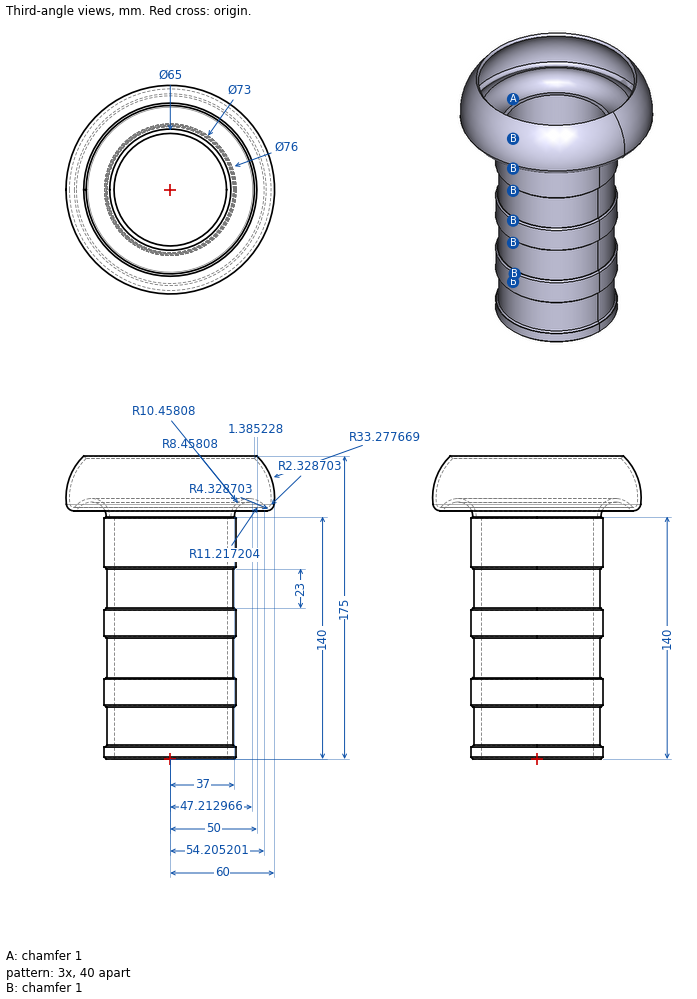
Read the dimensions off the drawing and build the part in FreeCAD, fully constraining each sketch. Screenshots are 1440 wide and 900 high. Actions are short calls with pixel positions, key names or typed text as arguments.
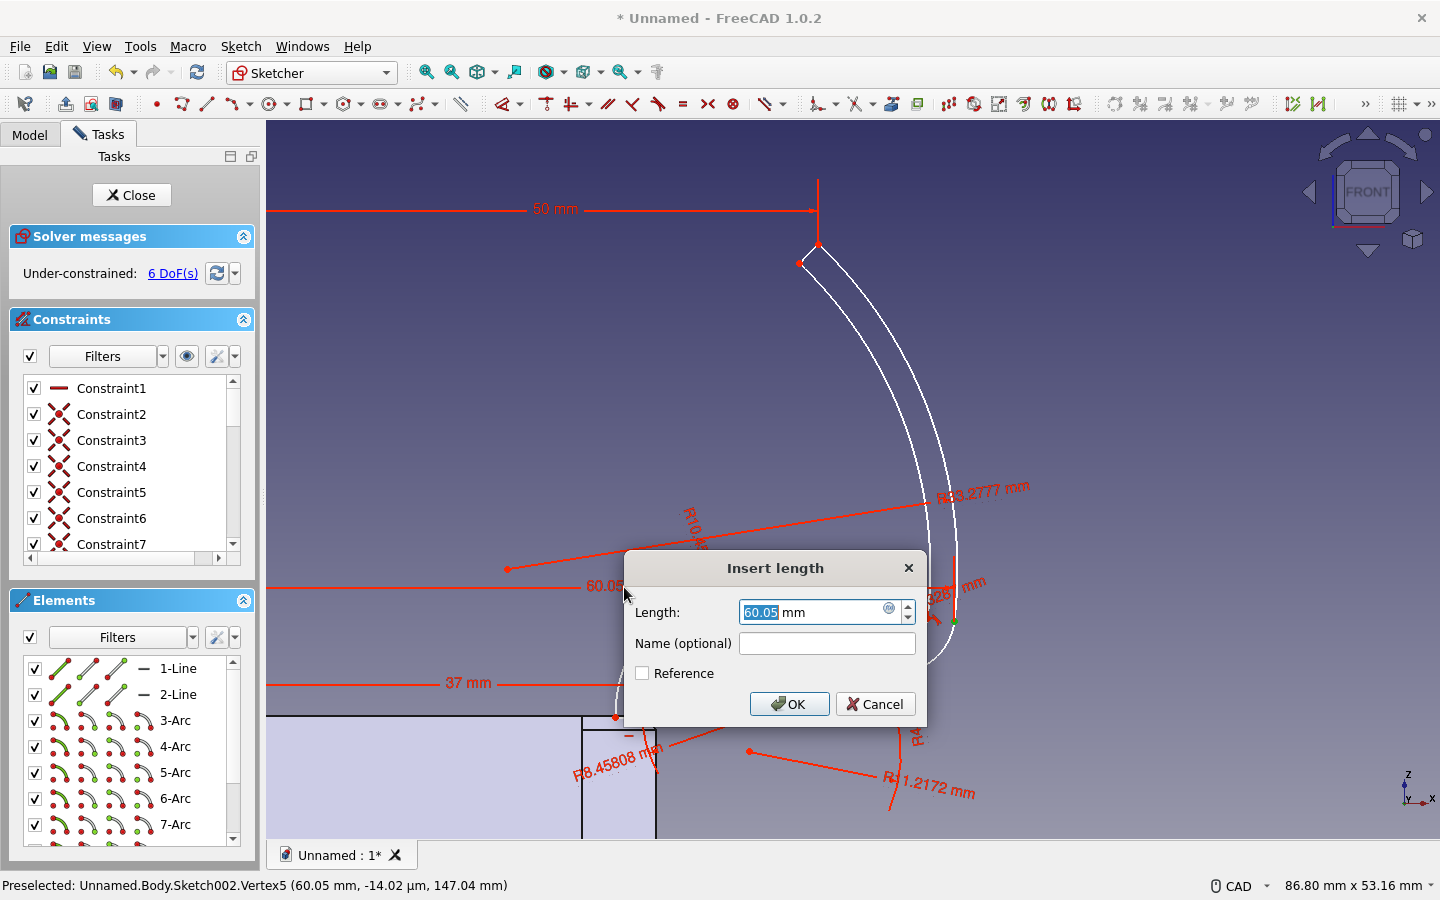
text(60)
key(Return)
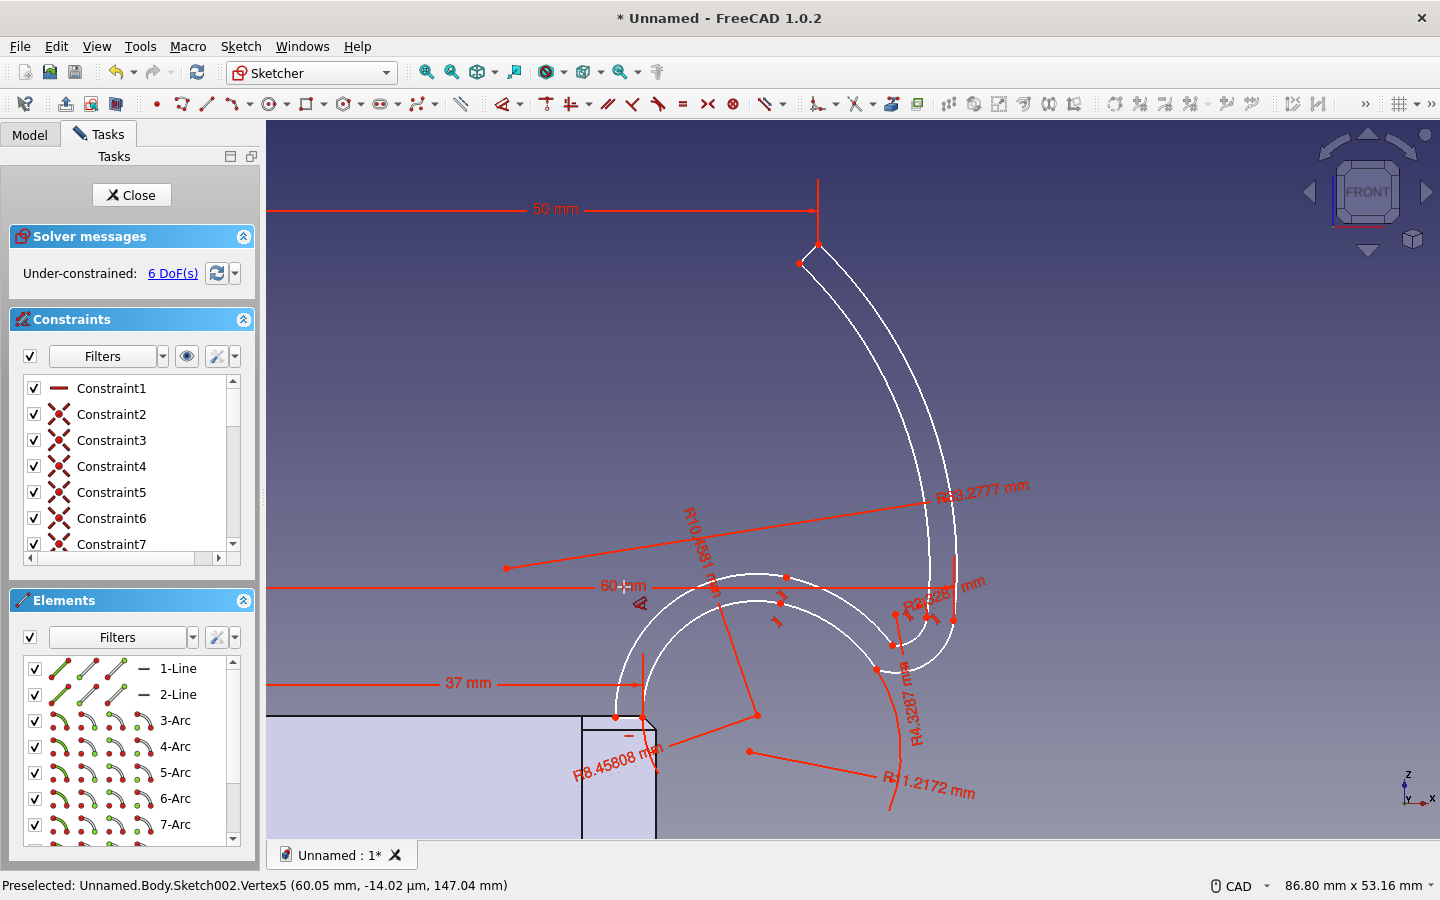
click(818, 244)
click(852, 528)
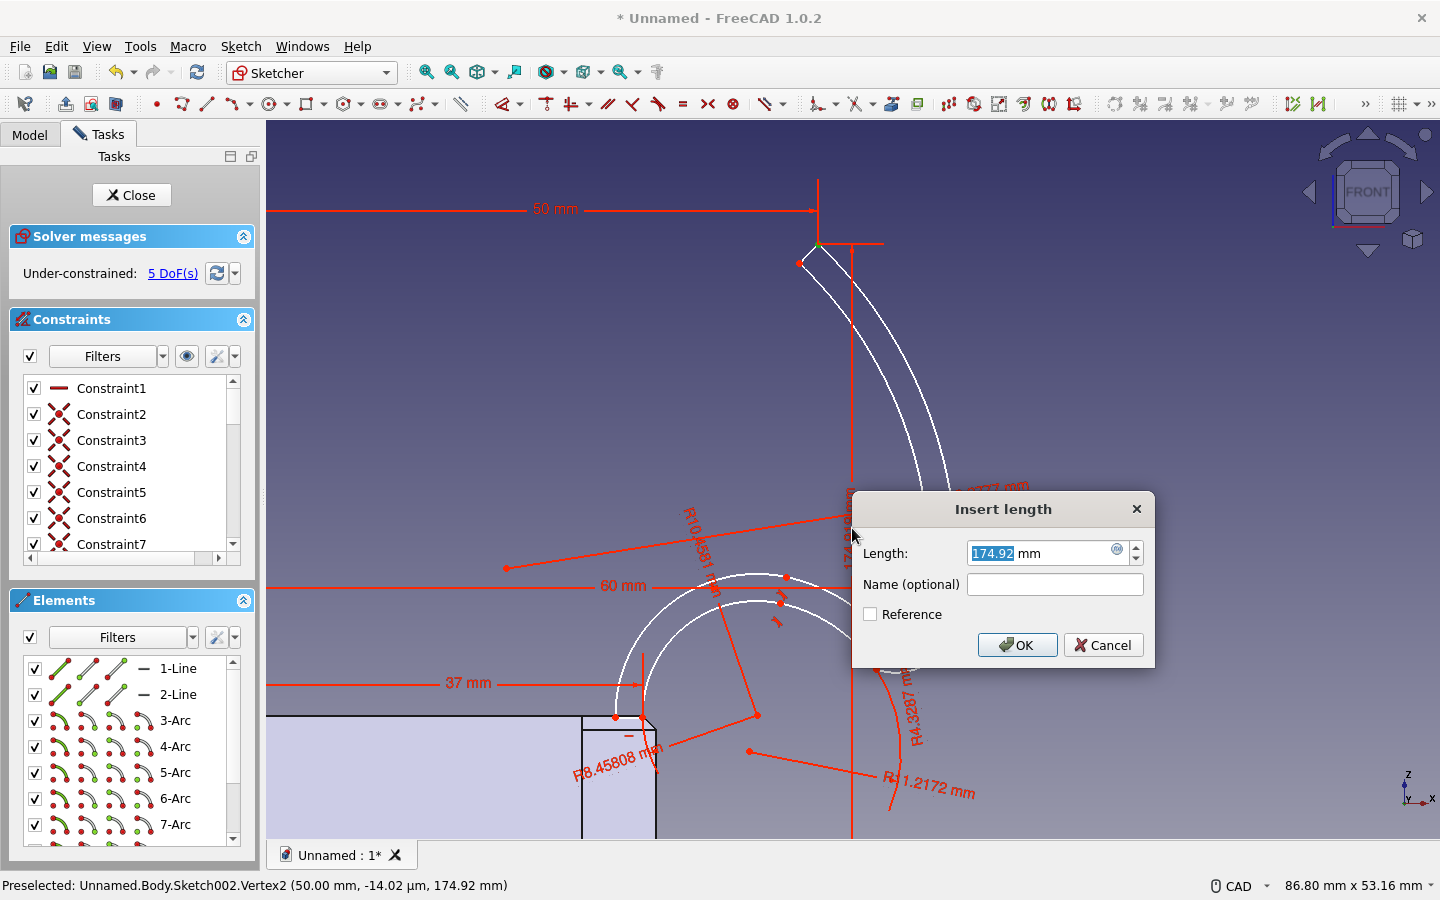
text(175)
key(Return)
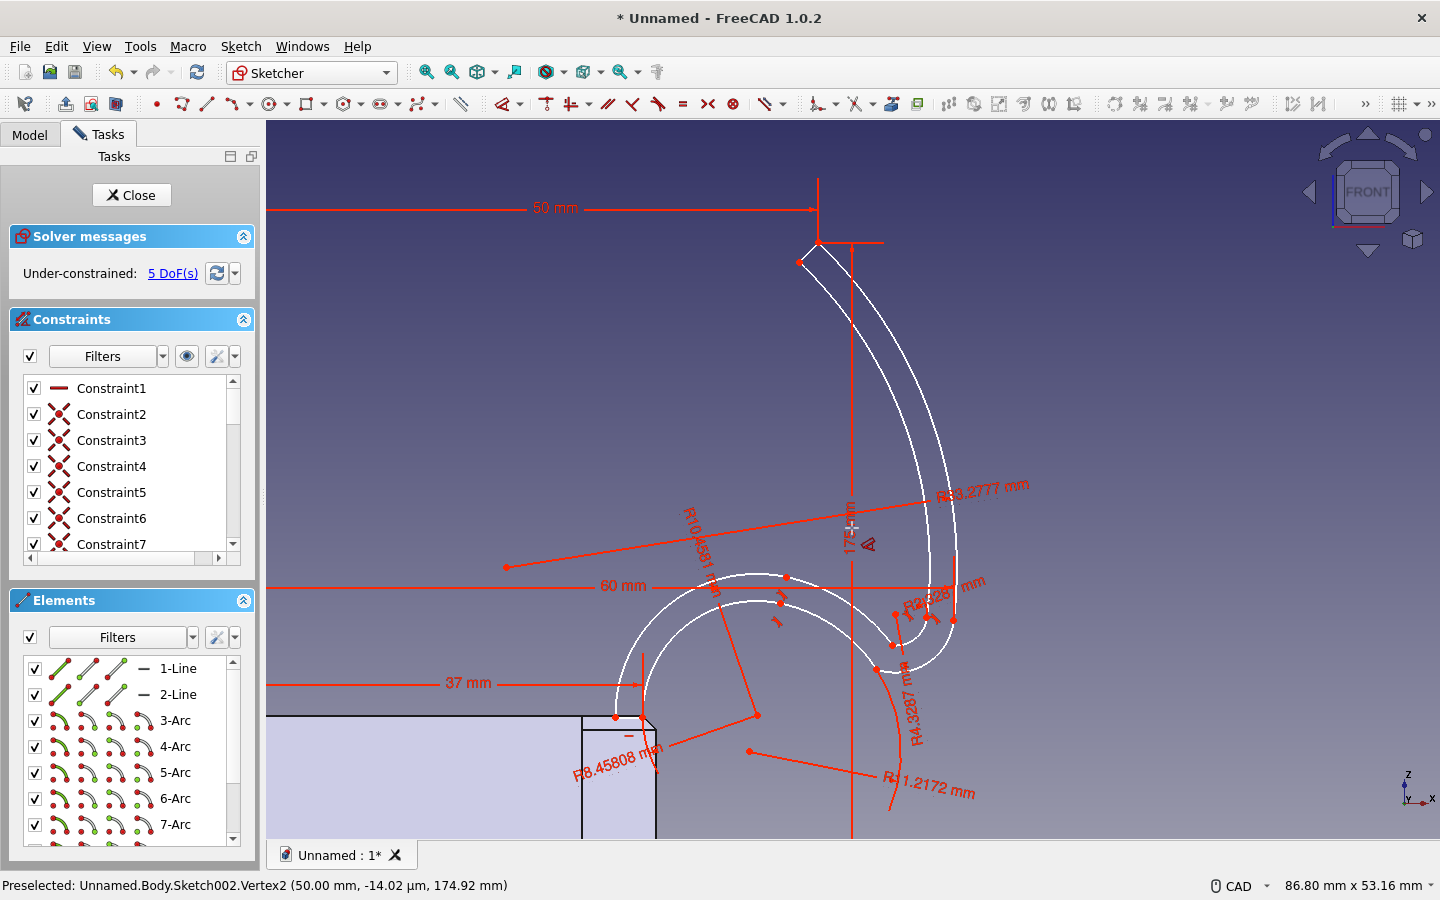
click(643, 718)
click(677, 743)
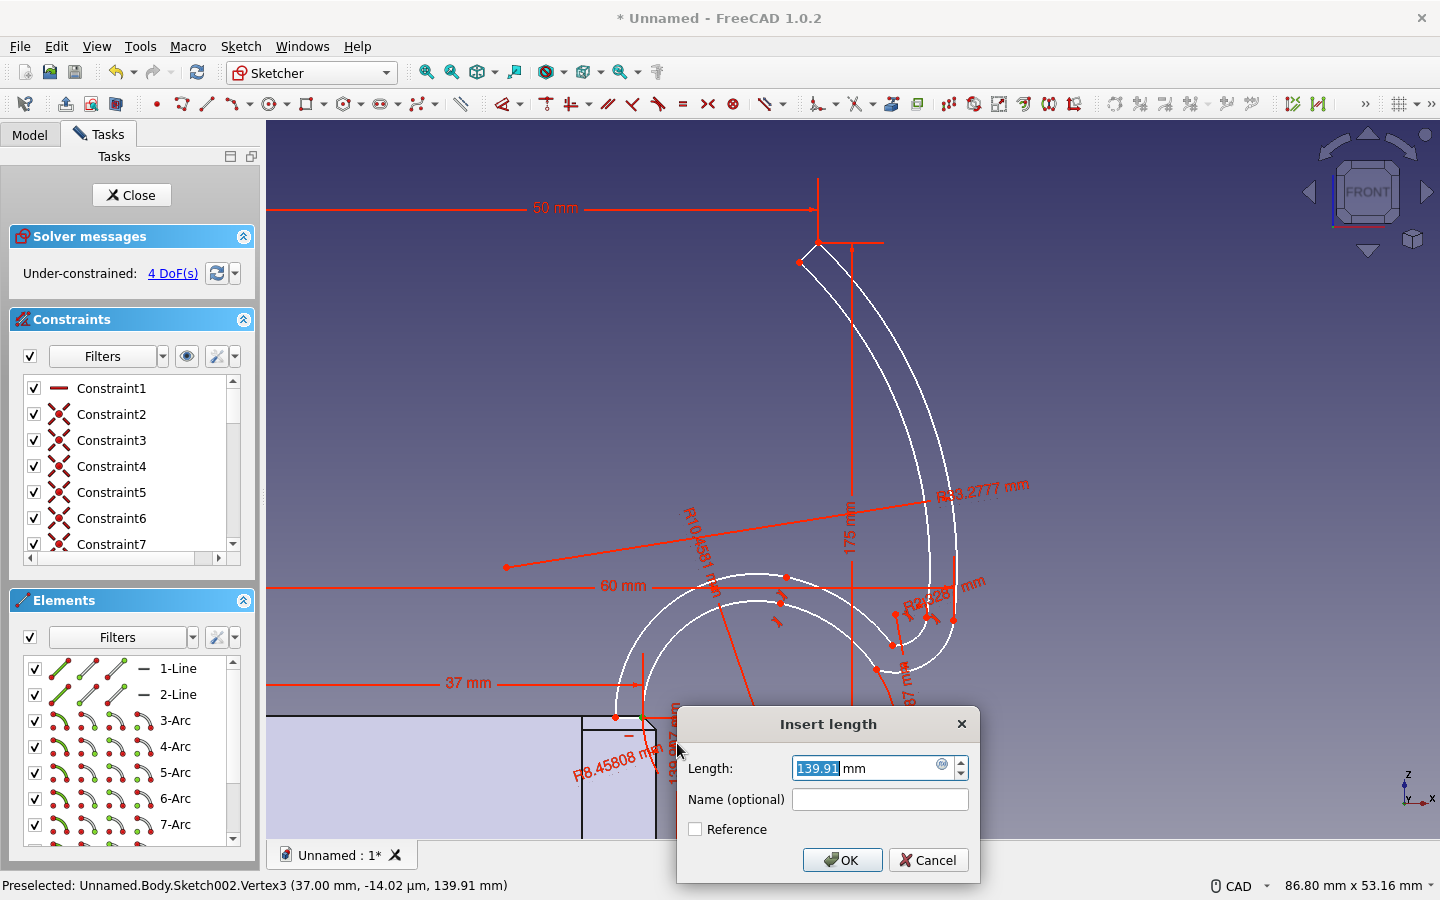
text(140)
key(Return)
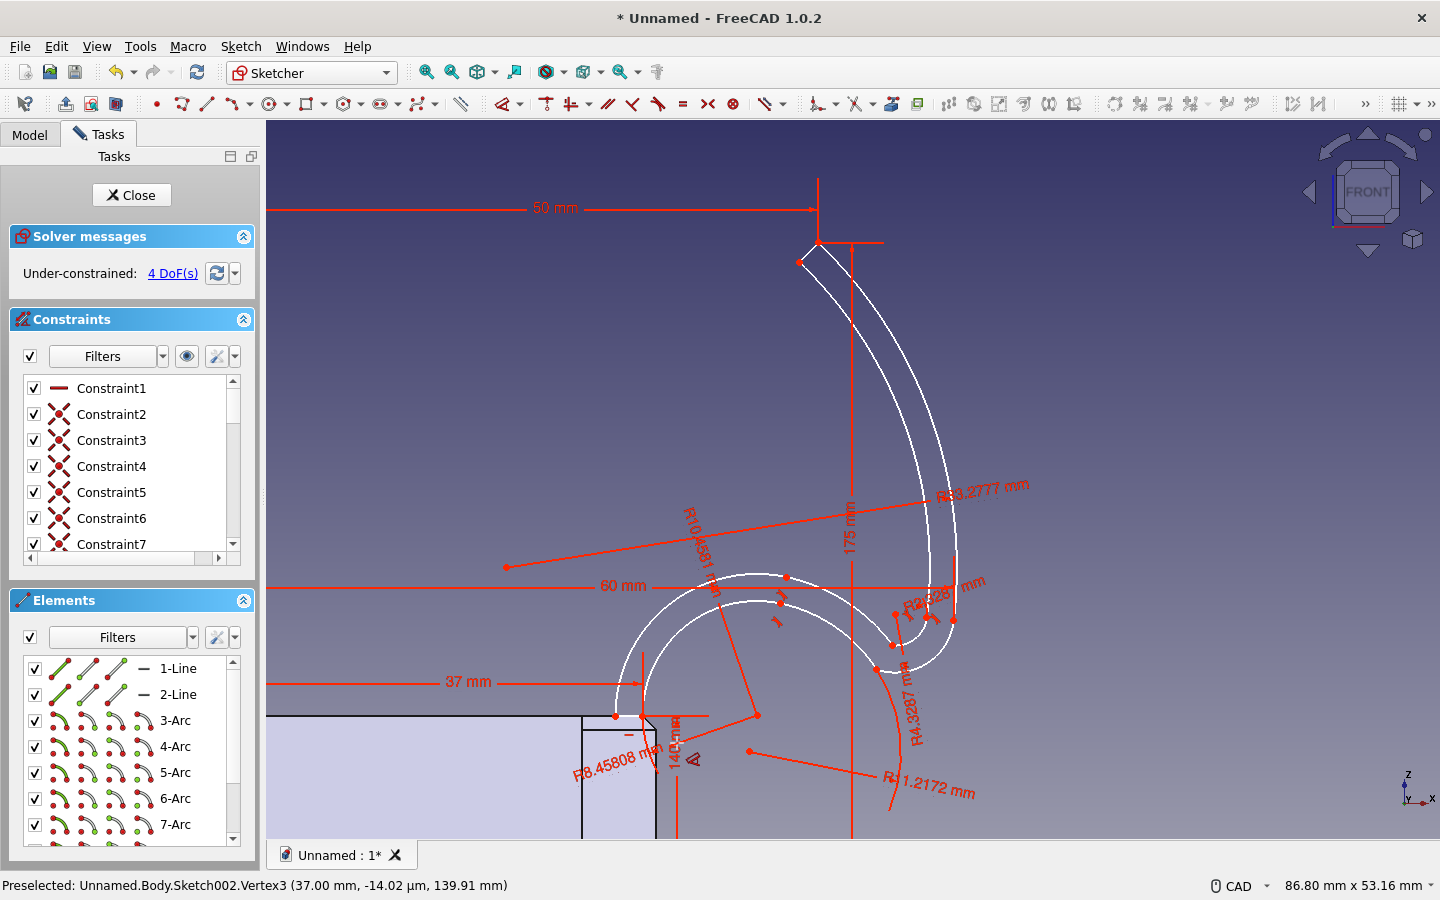
click(757, 715)
click(791, 763)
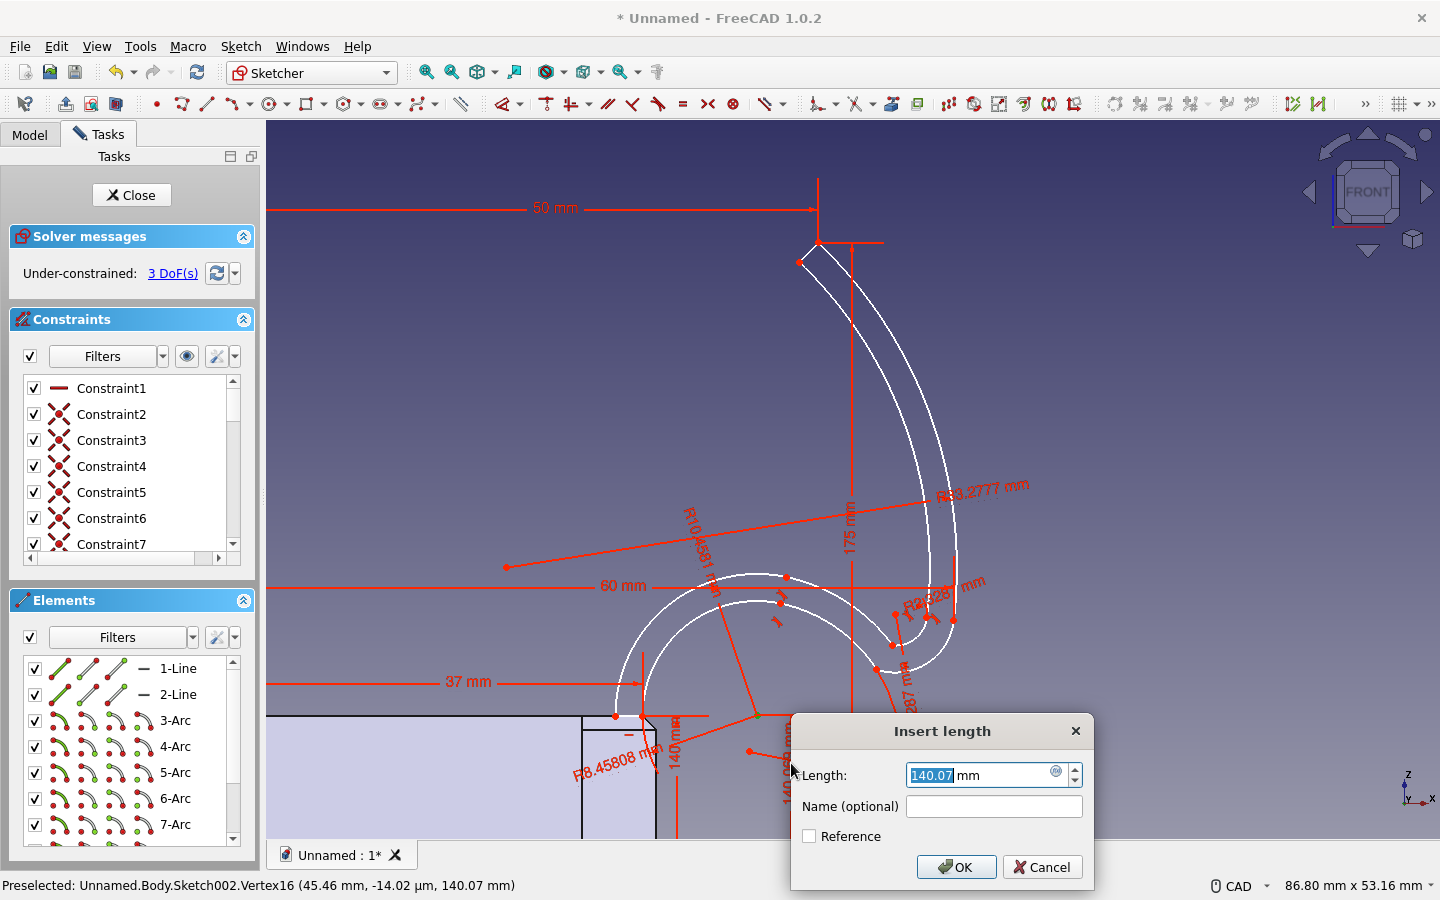
text(140)
key(Return)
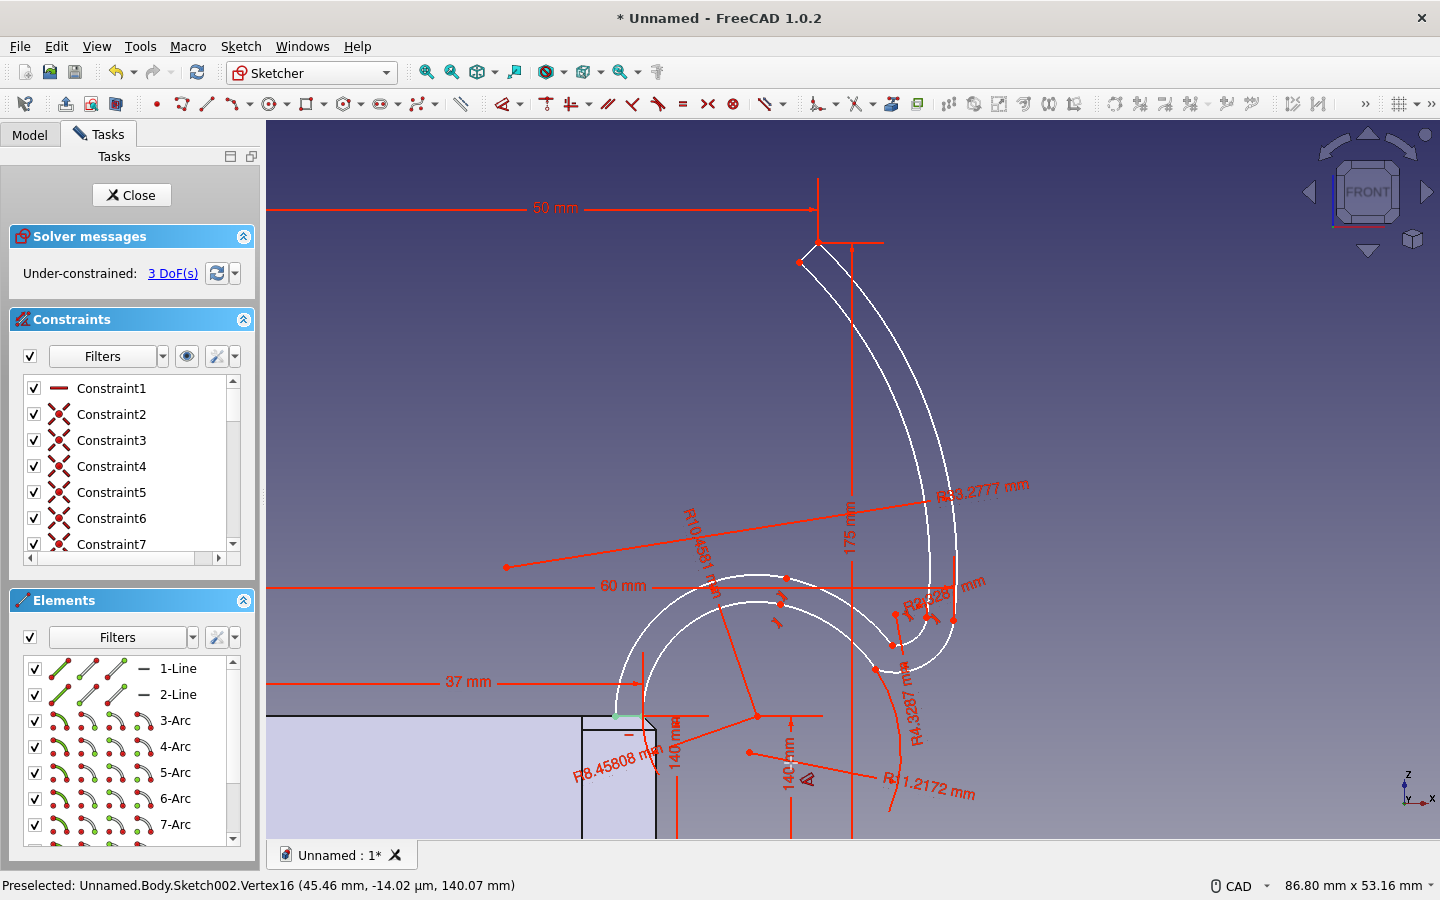
scroll(807, 255, up, 4)